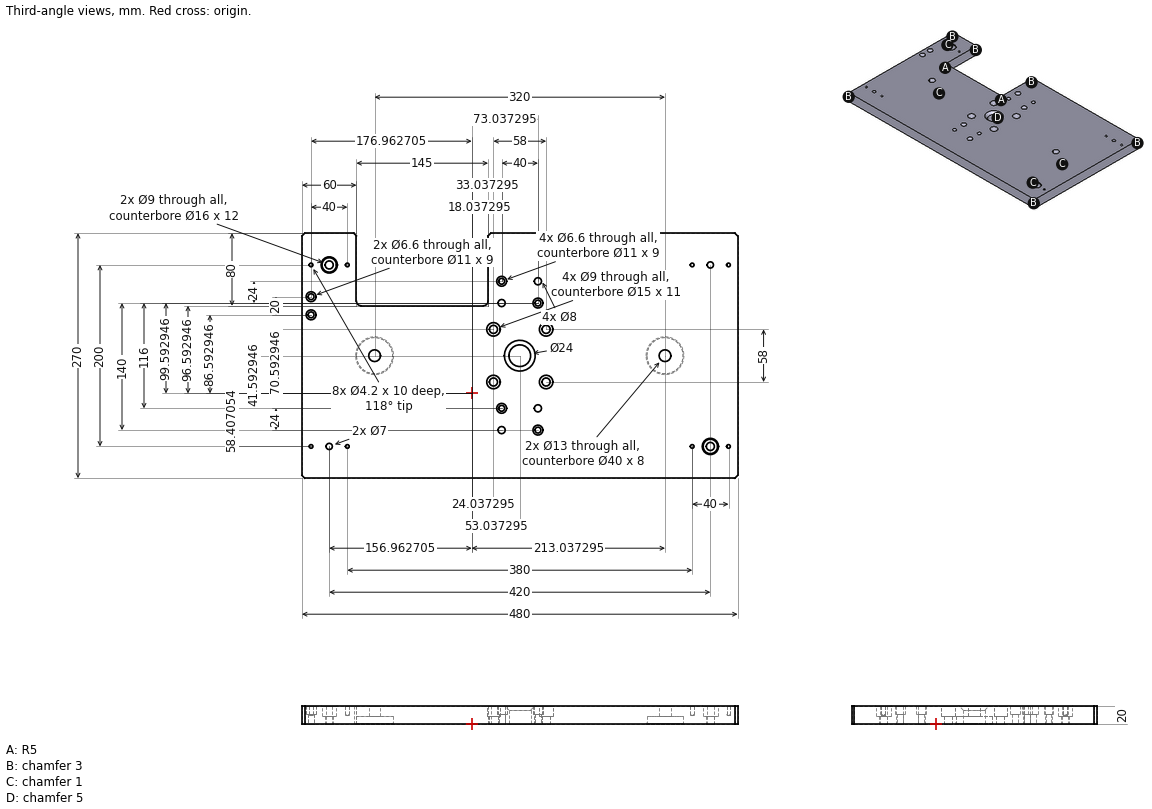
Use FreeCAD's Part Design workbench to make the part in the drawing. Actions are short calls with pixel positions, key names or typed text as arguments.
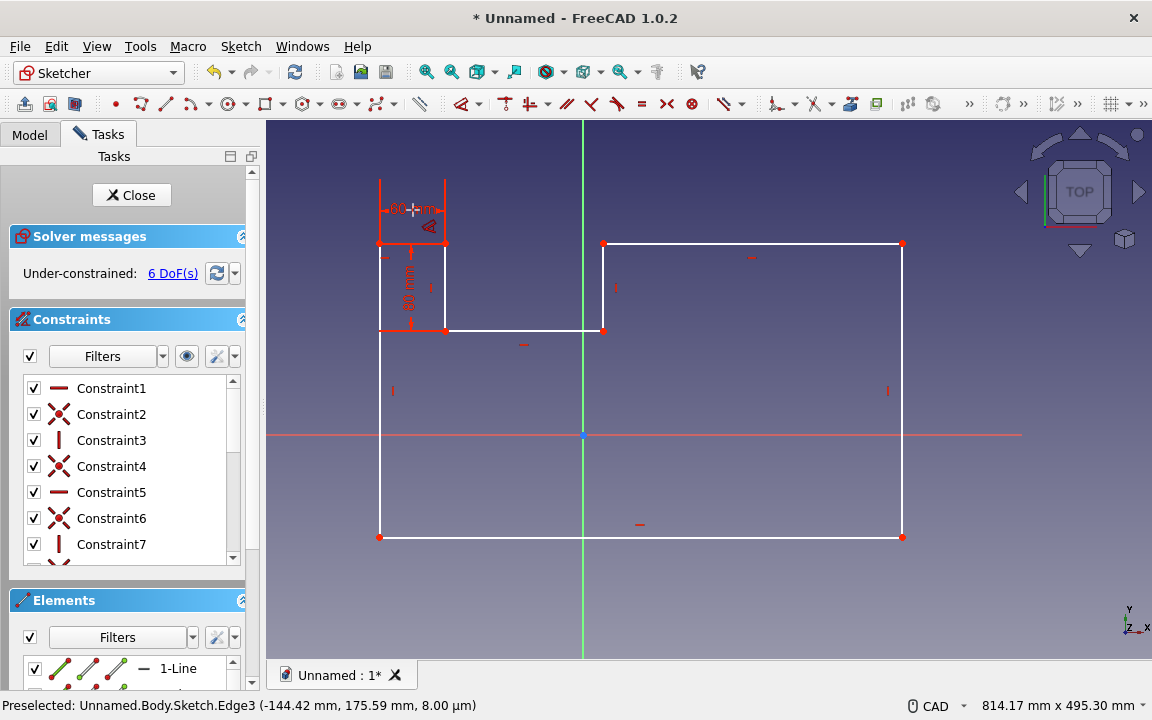
click(603, 270)
click(569, 288)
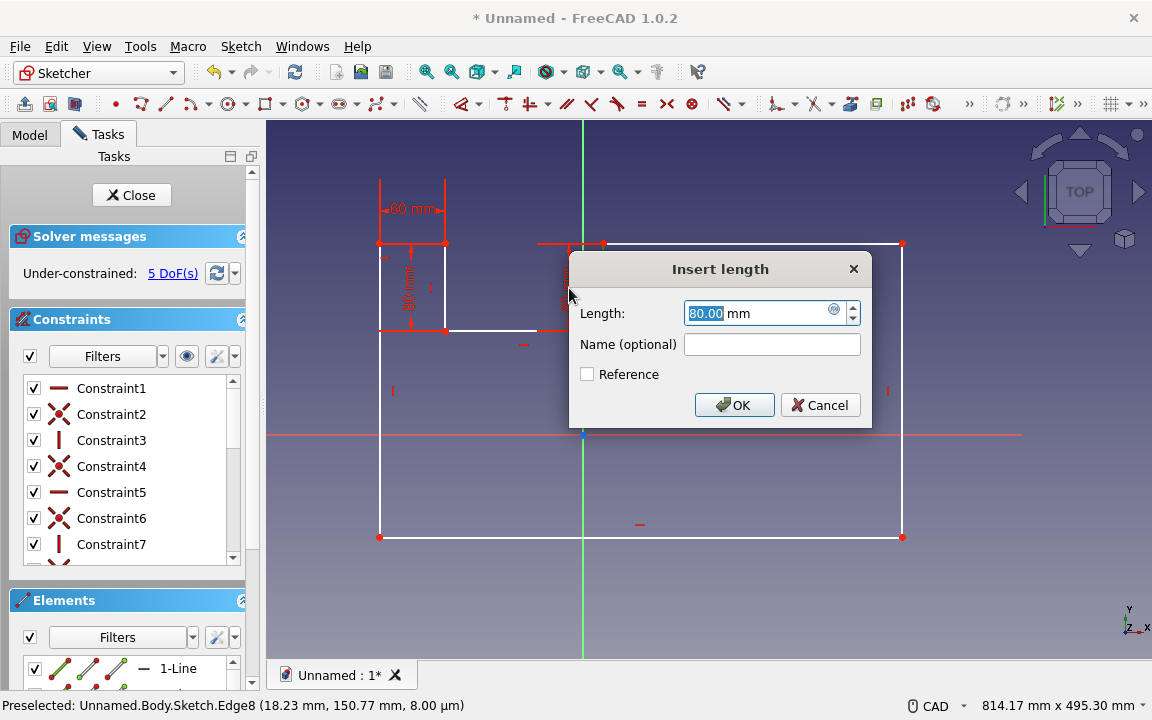
text(80)
key(Return)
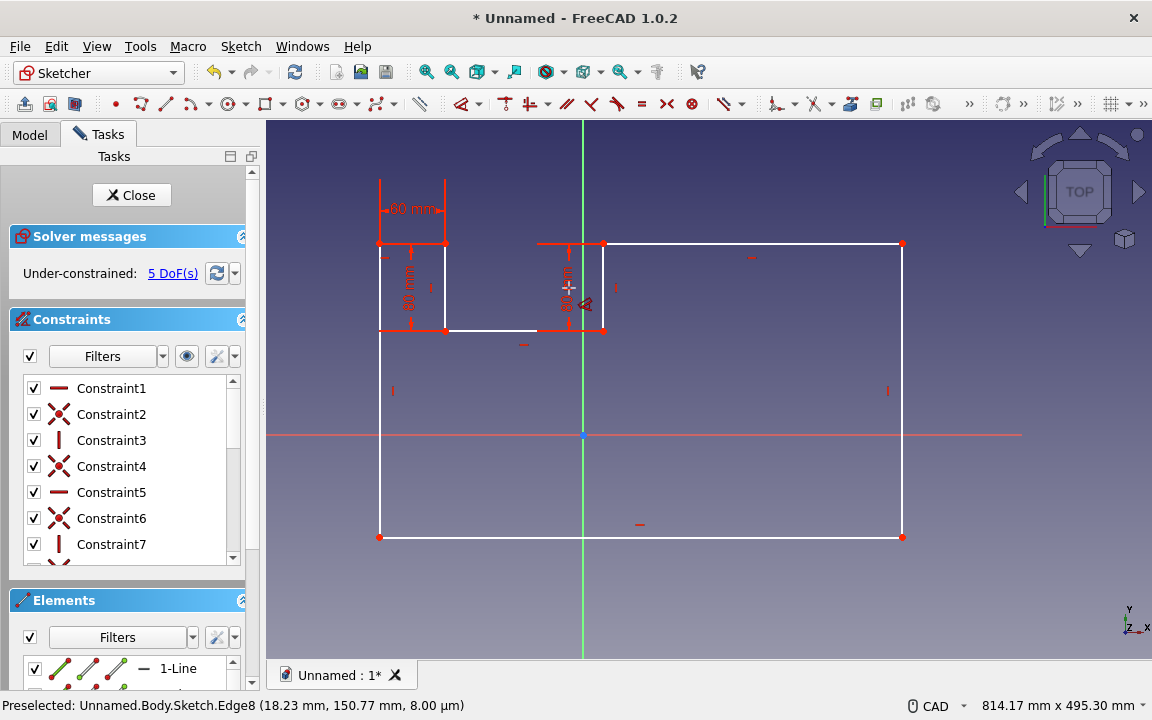
click(556, 331)
click(488, 297)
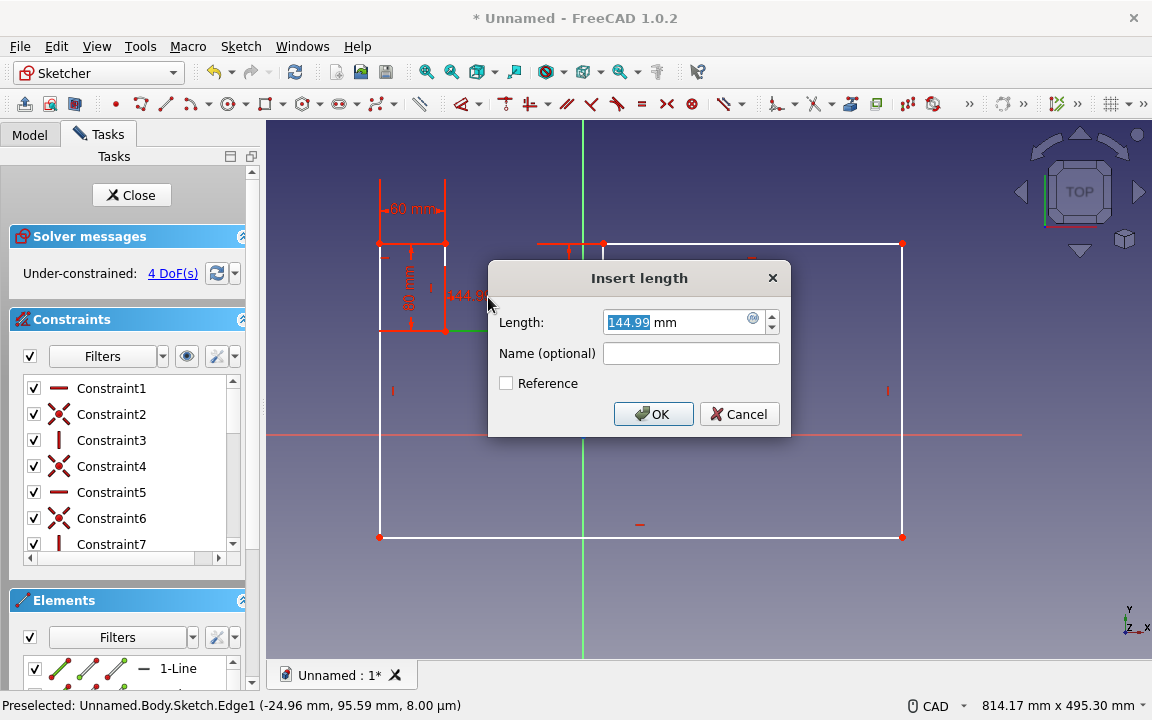
text(145)
key(Return)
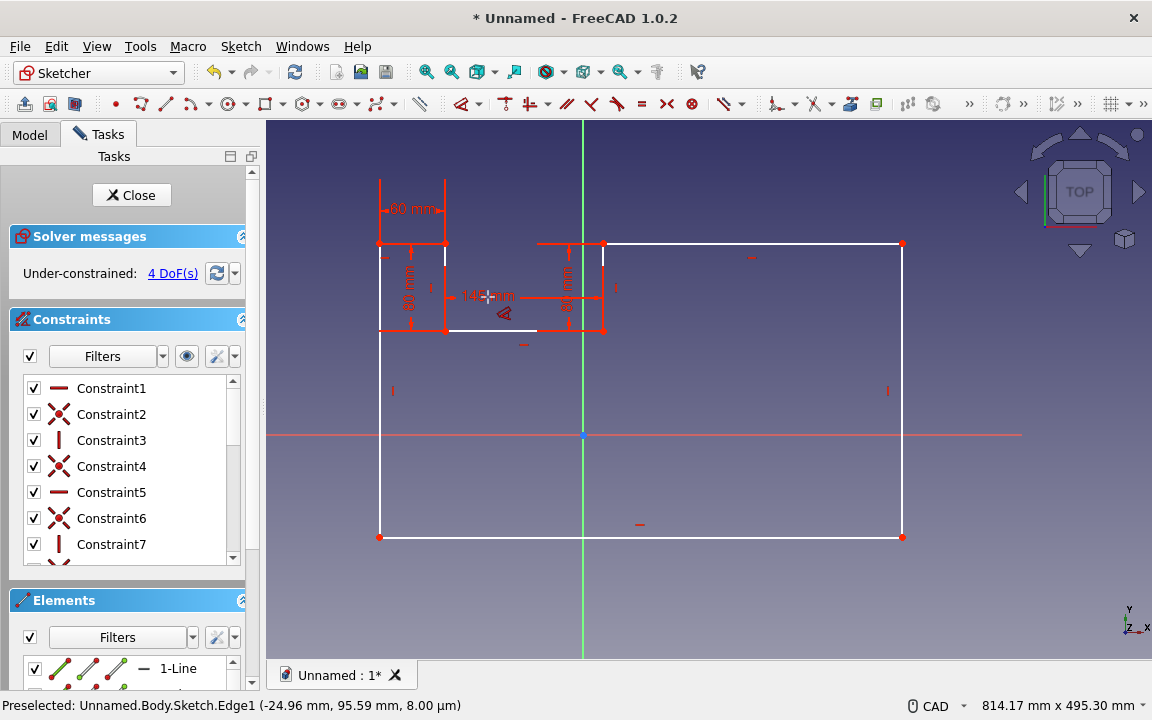
click(380, 332)
click(346, 391)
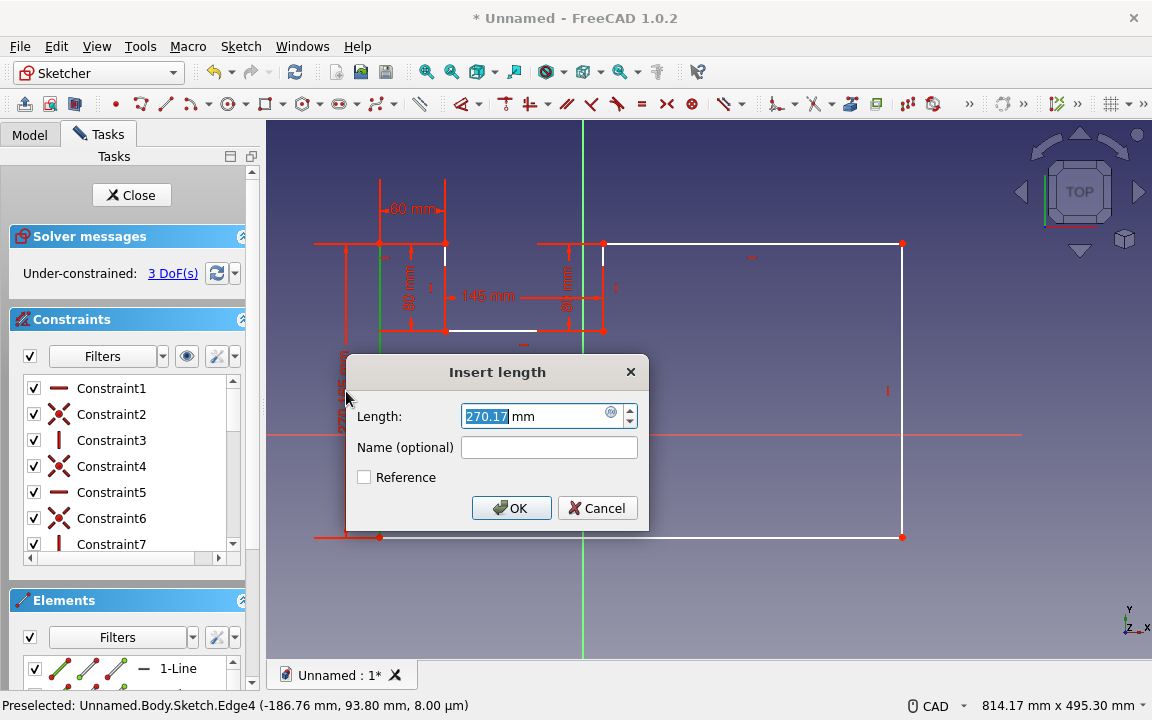
text(270)
key(Return)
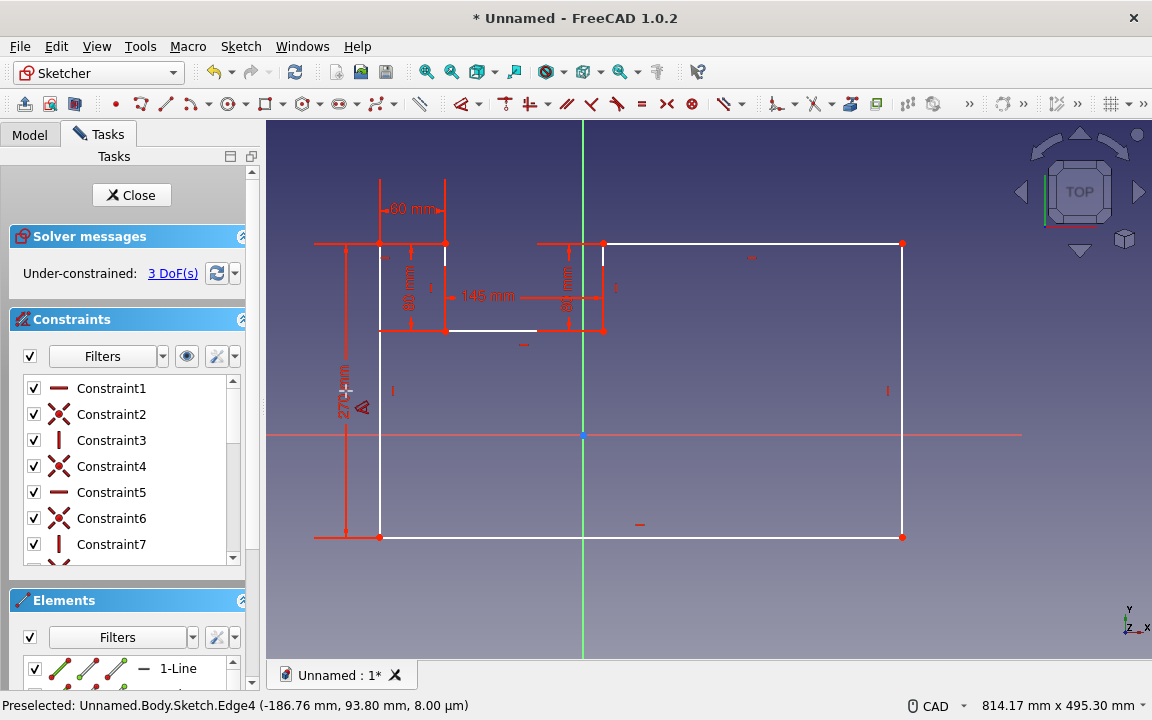
click(537, 538)
click(641, 572)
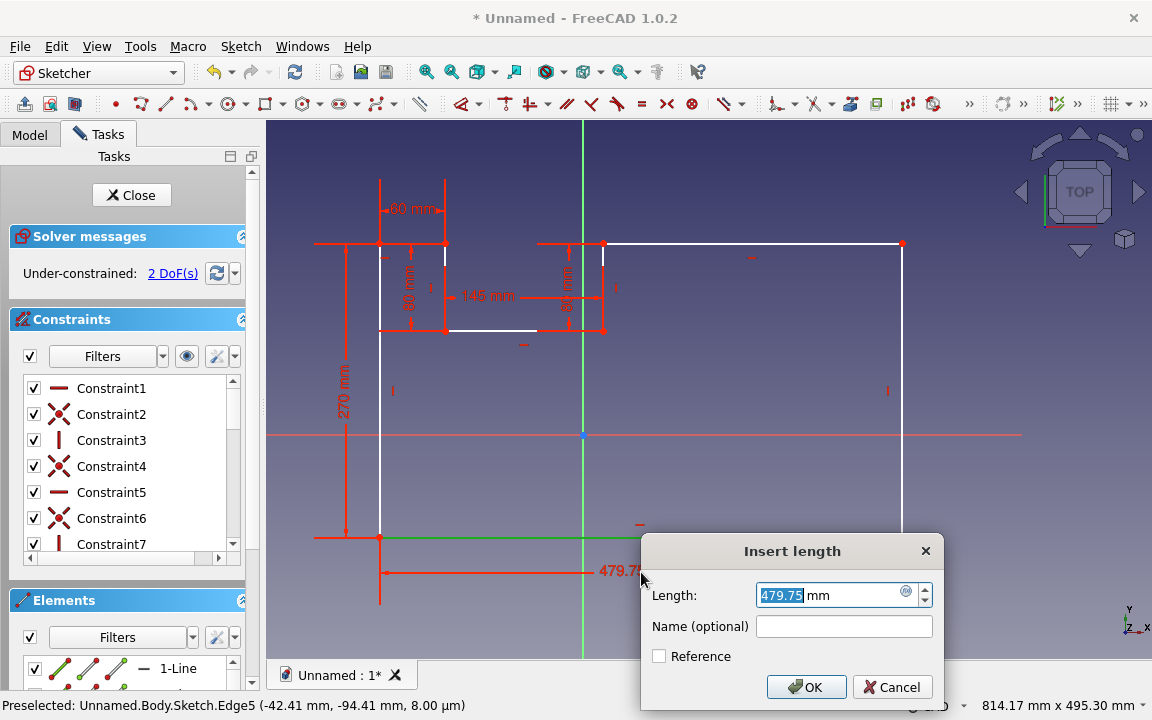
text(480)
key(Return)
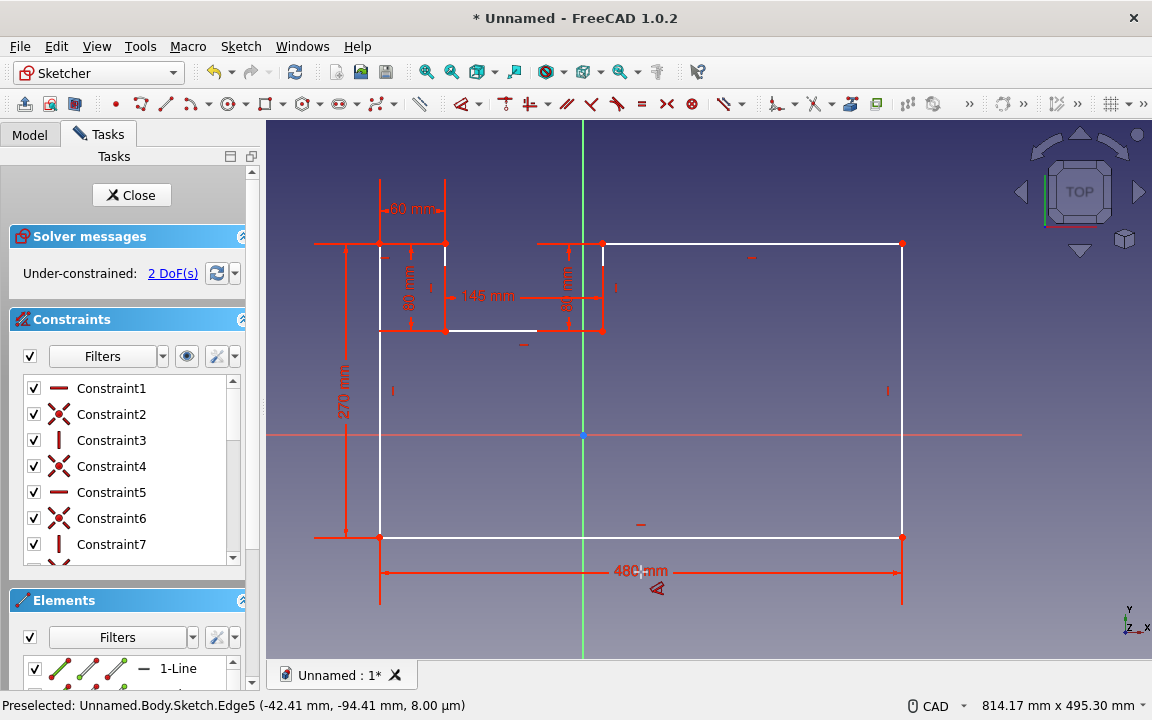
scroll(603, 331, up, 4)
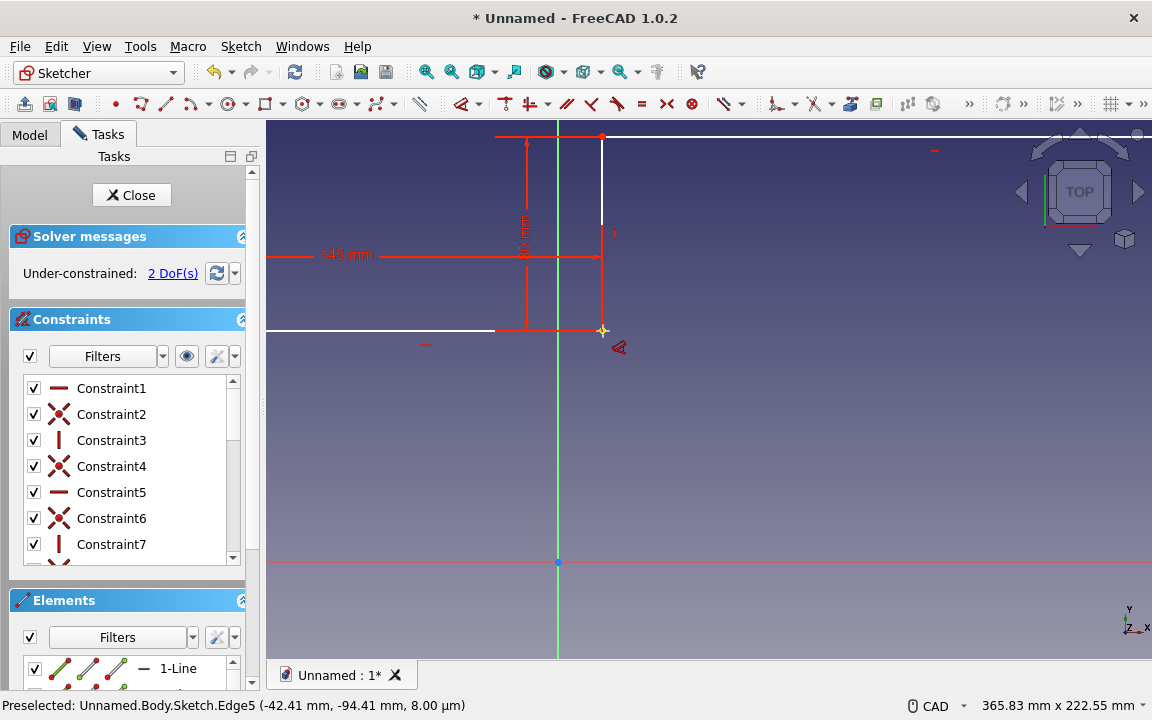
click(602, 331)
click(580, 297)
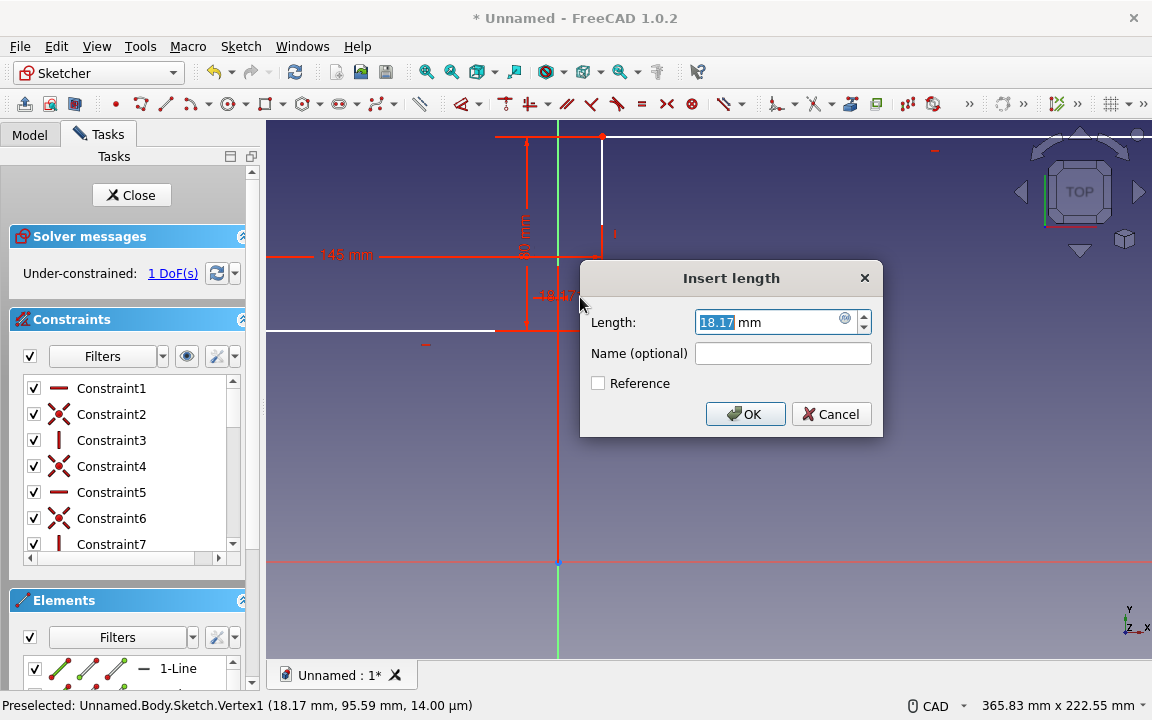
text(18.037295)
key(Return)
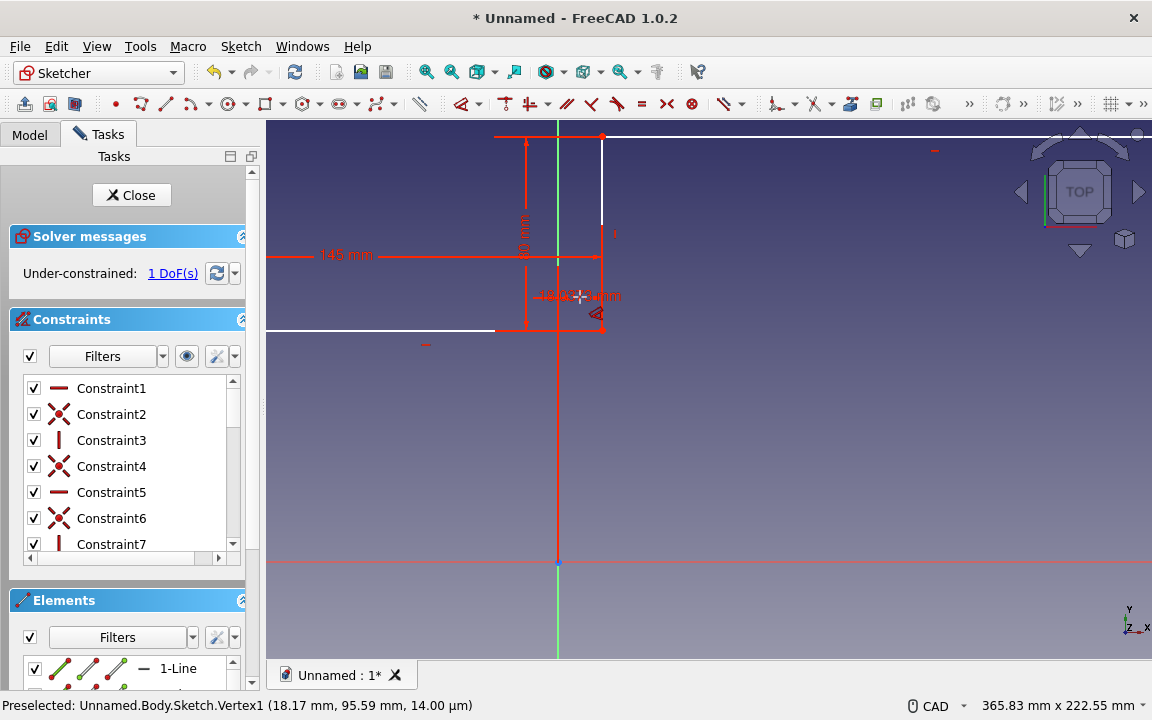
click(602, 331)
click(524, 446)